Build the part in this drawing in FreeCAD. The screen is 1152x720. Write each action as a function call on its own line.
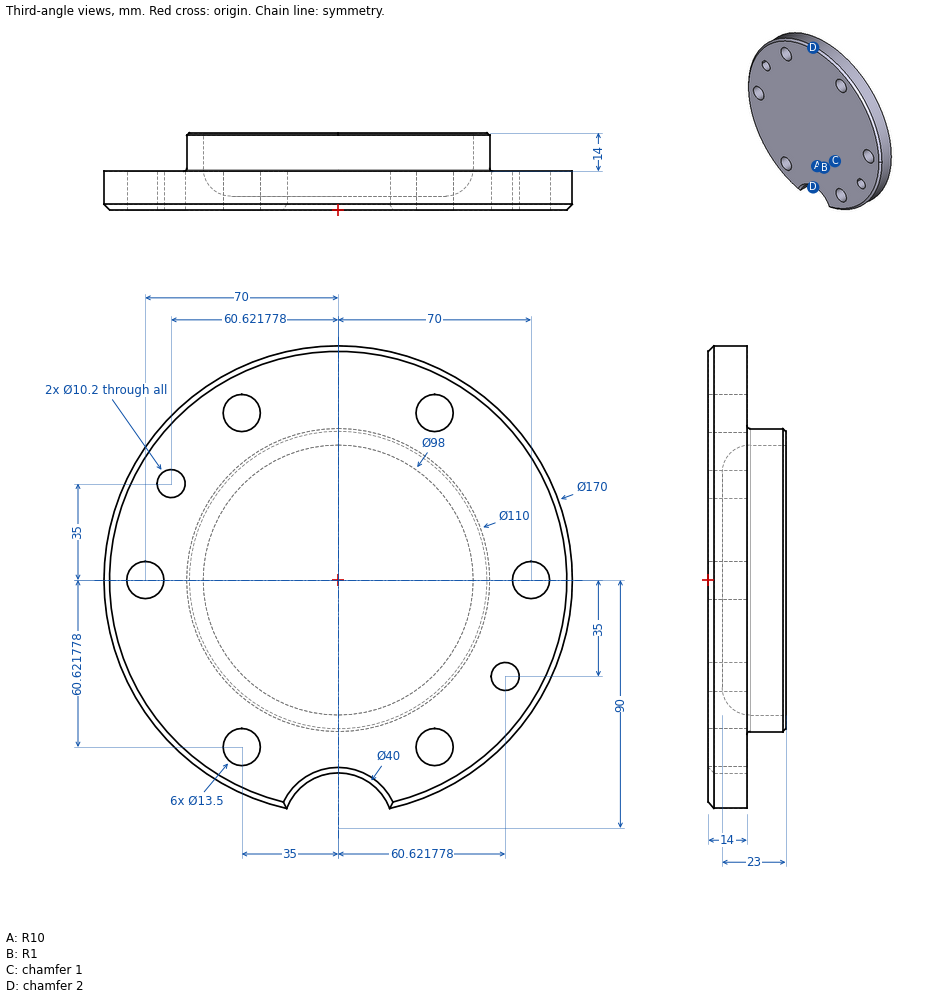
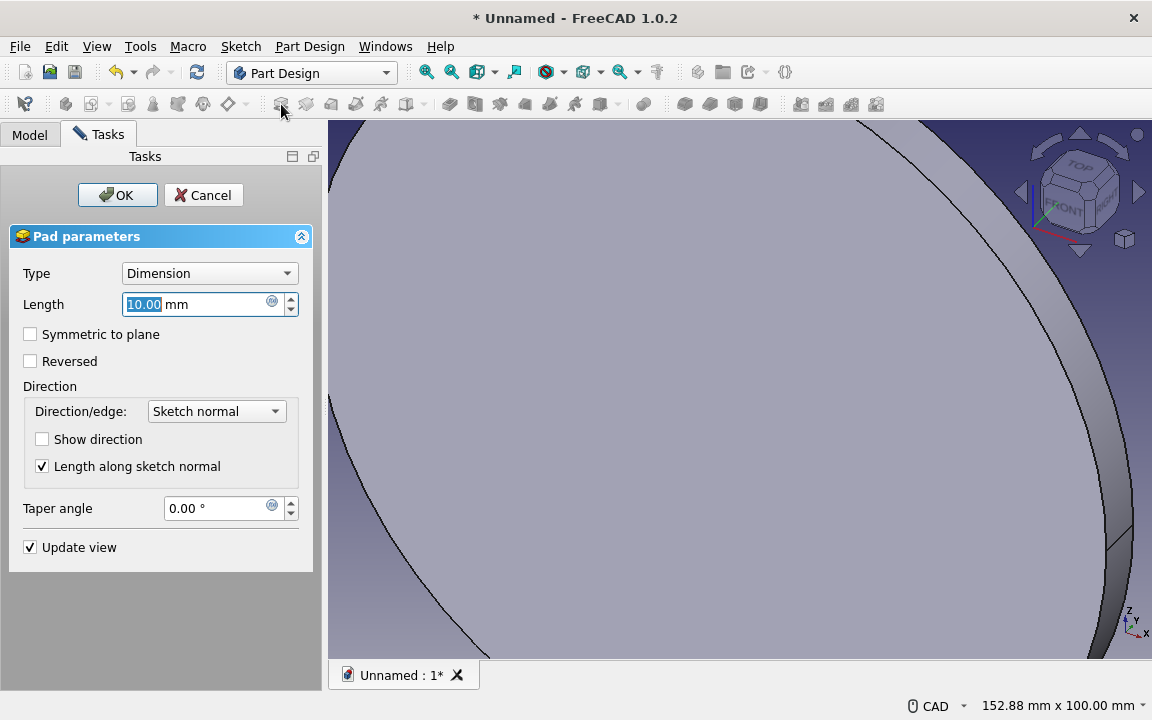
text(14)
key(Tab)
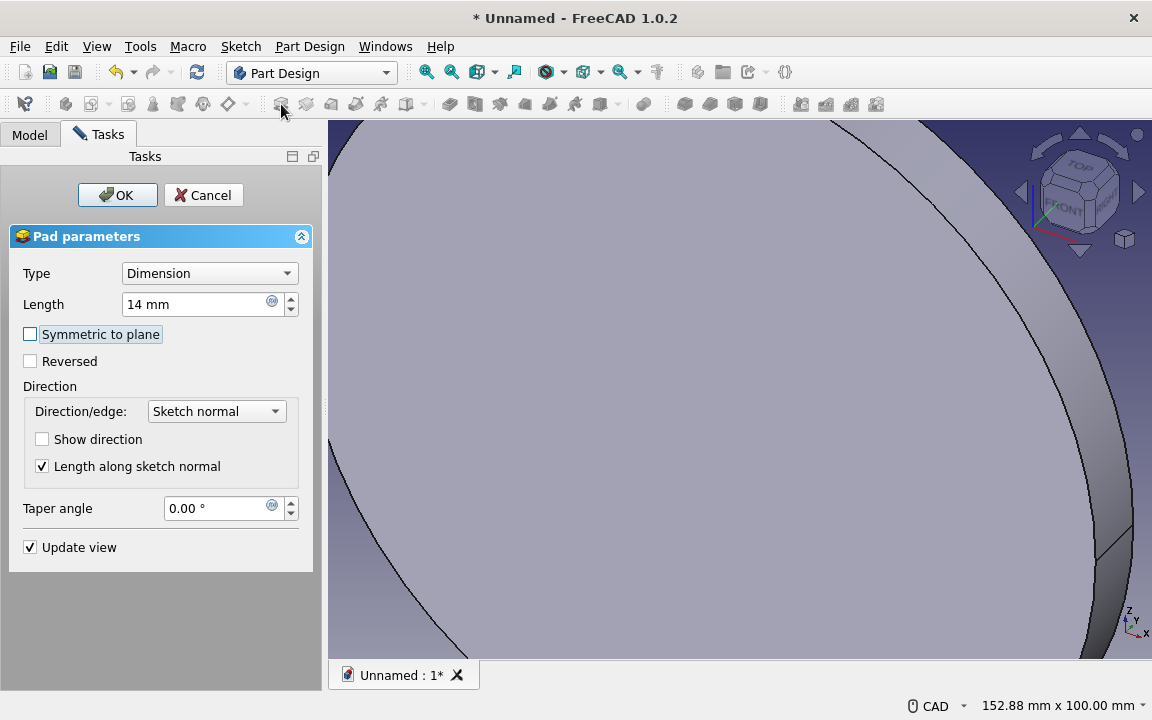
click(31, 361)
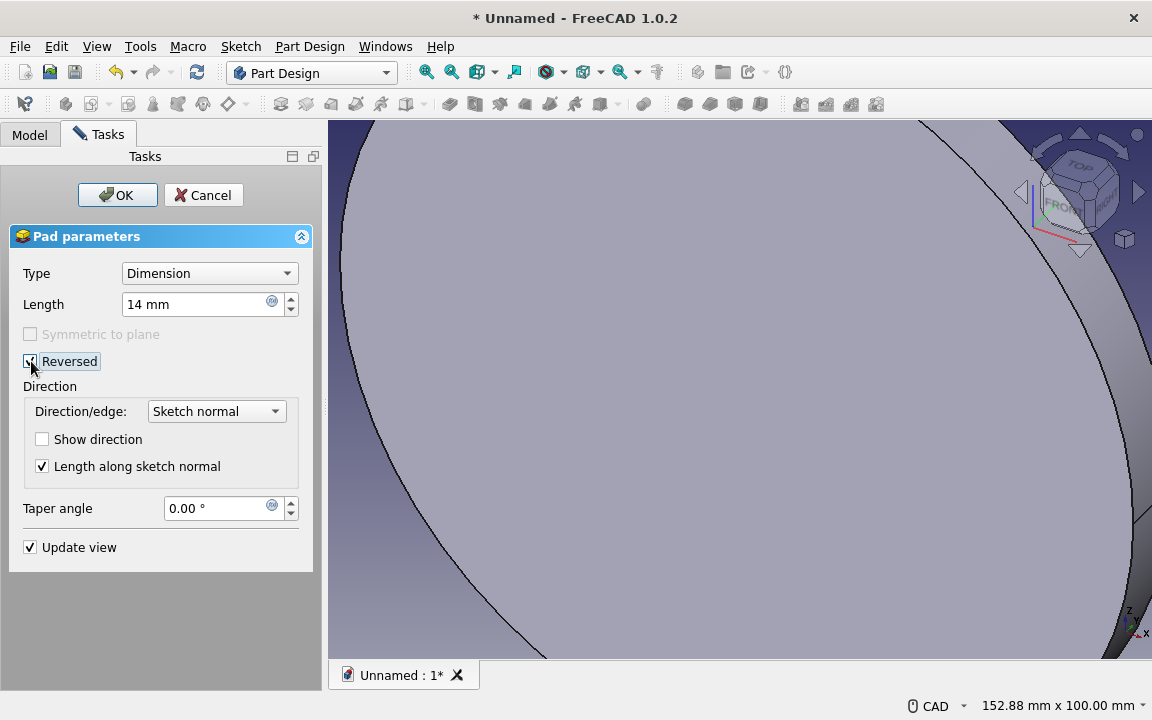
click(118, 195)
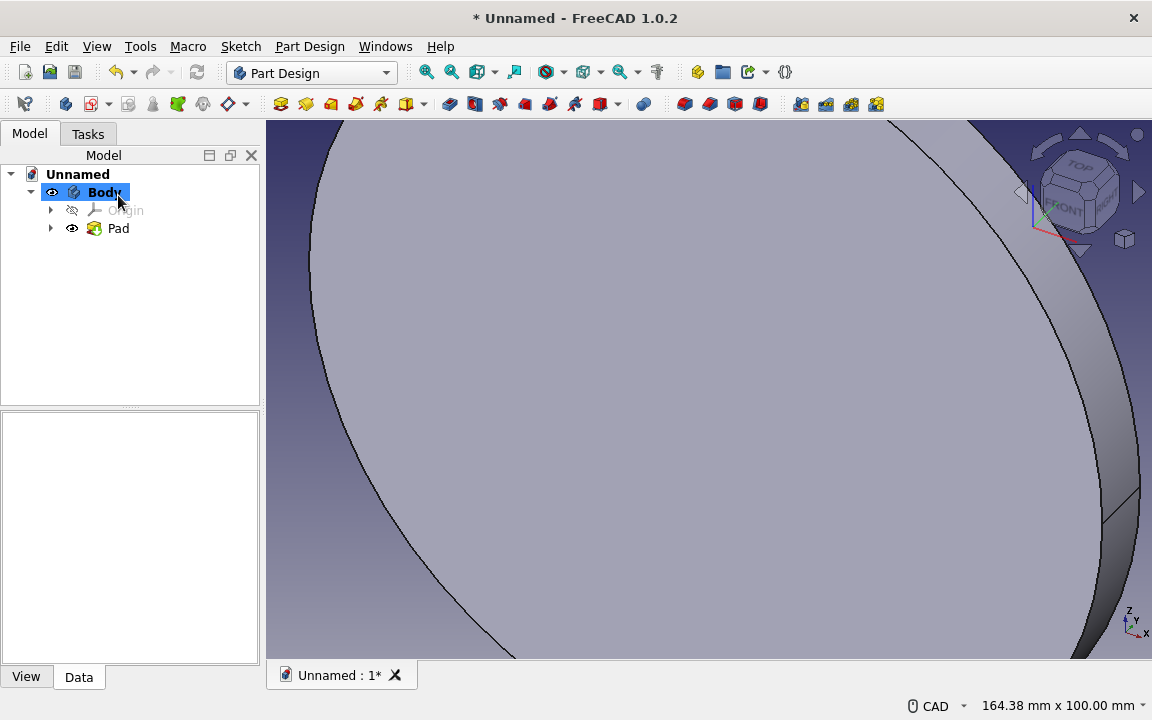
click(427, 72)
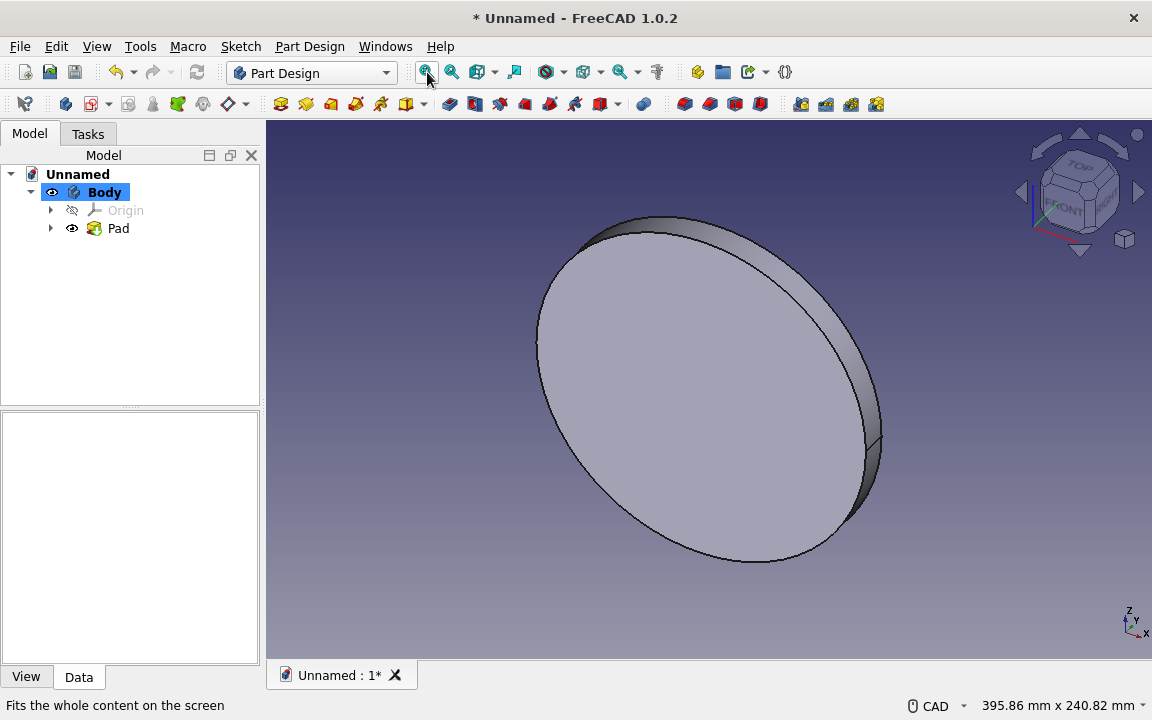
key(4)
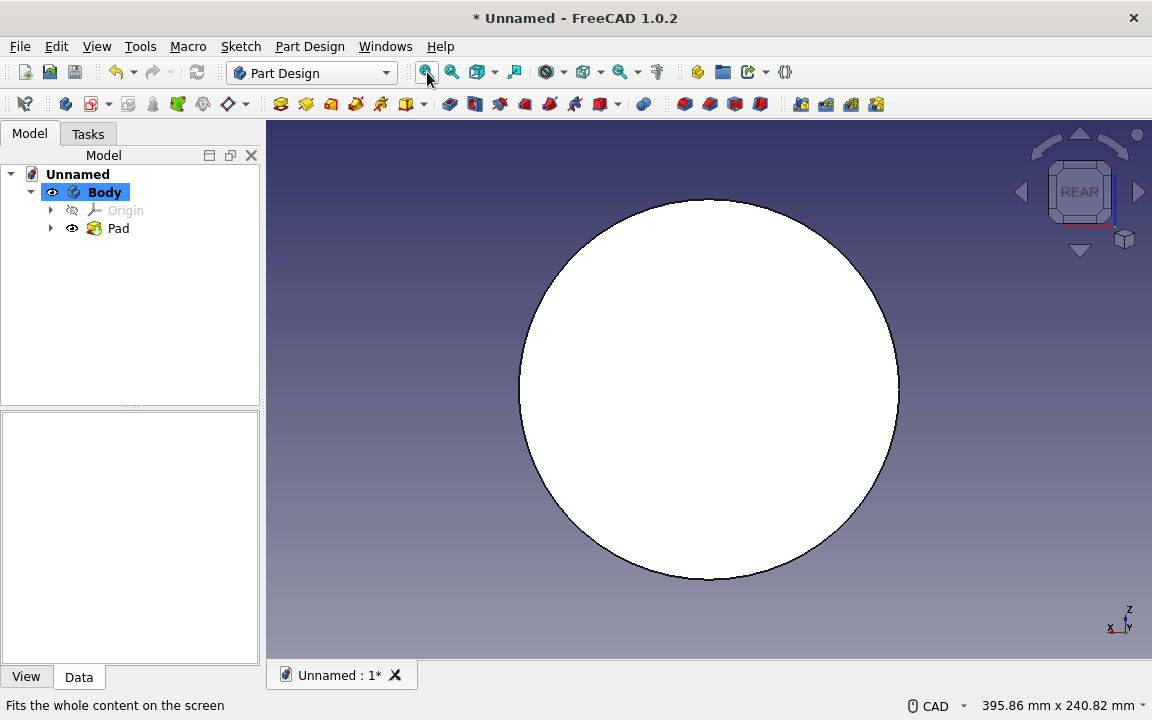
click(709, 388)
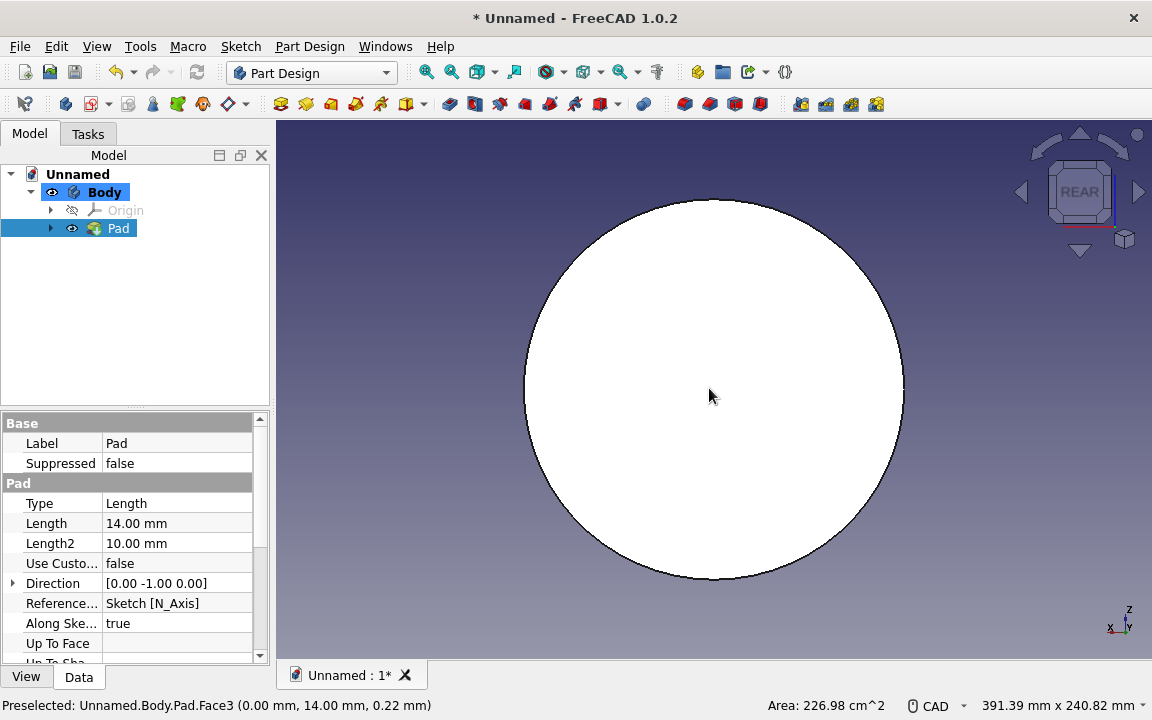
click(90, 104)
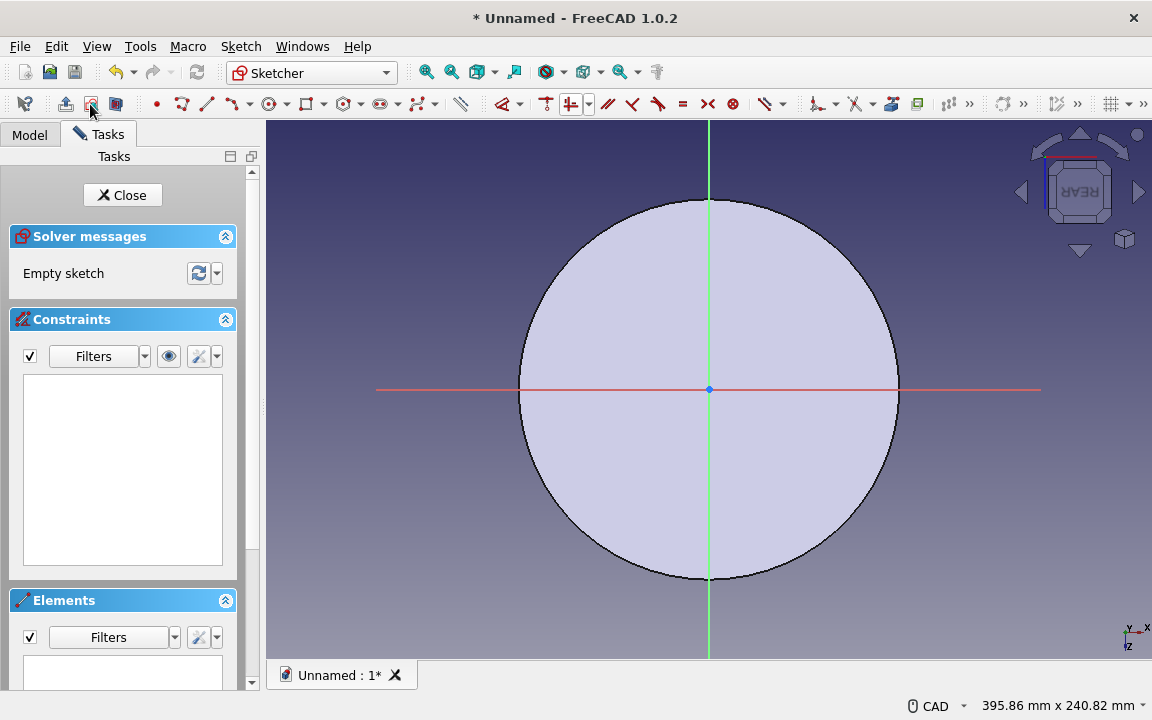
scroll(848, 390, up, 2)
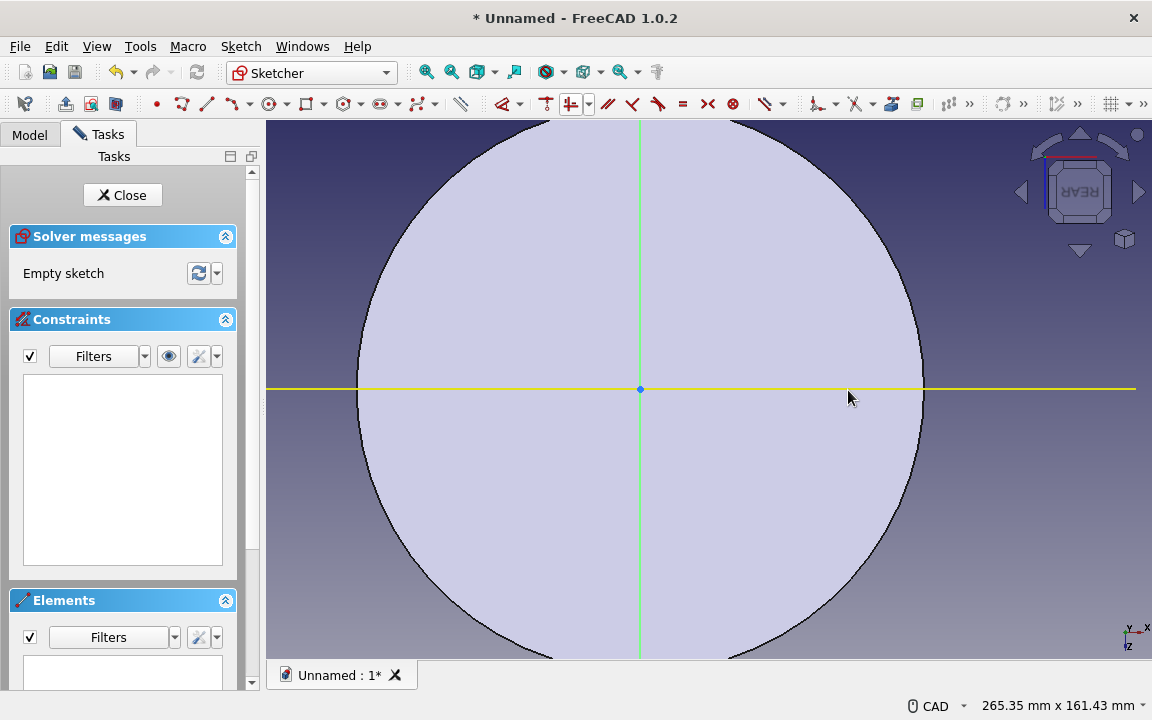
click(268, 104)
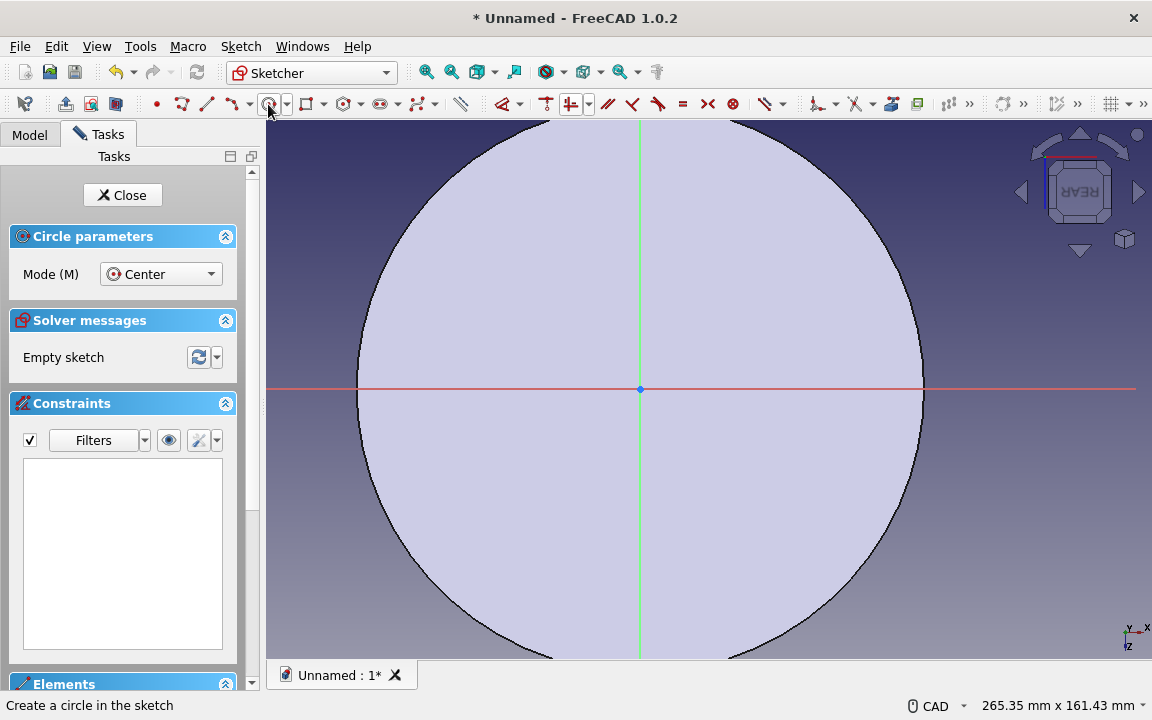
click(640, 389)
click(770, 259)
key(Escape)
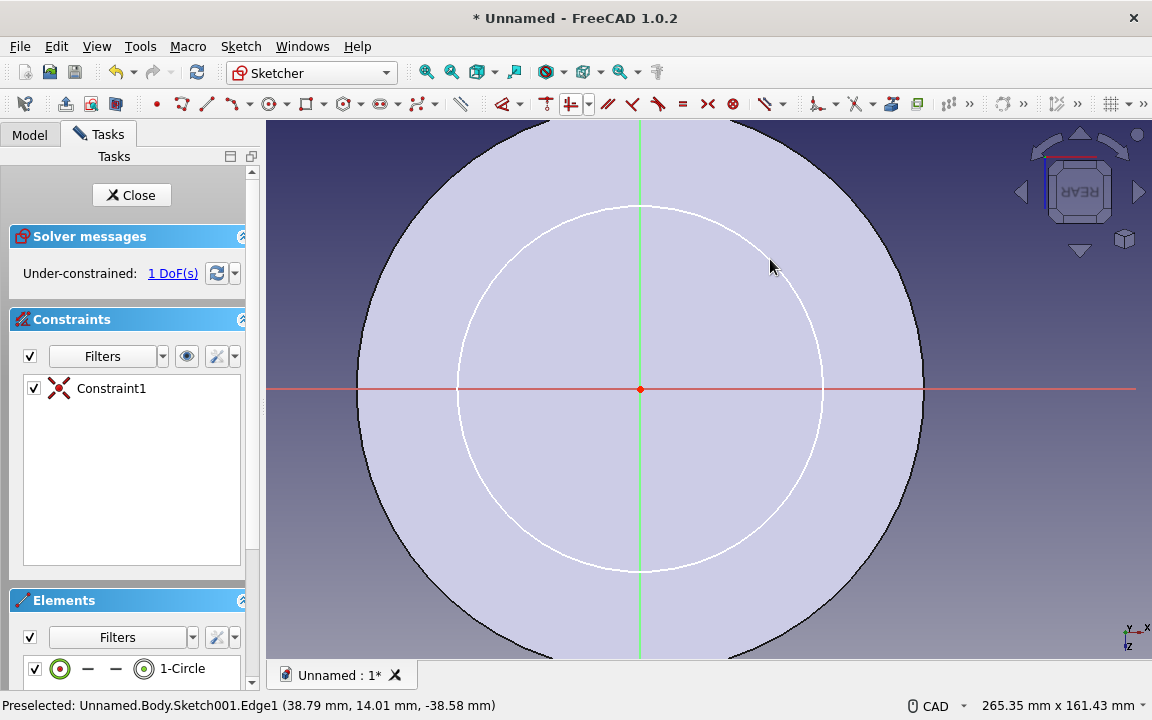
click(769, 259)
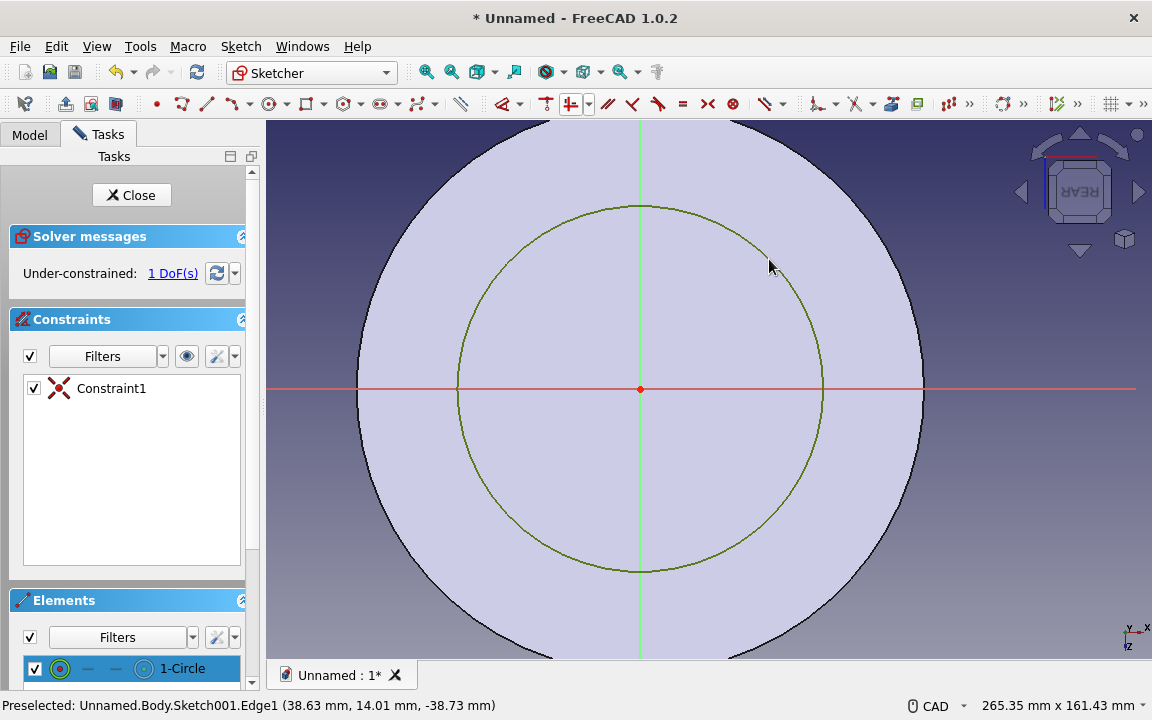
key(k)
key(o)